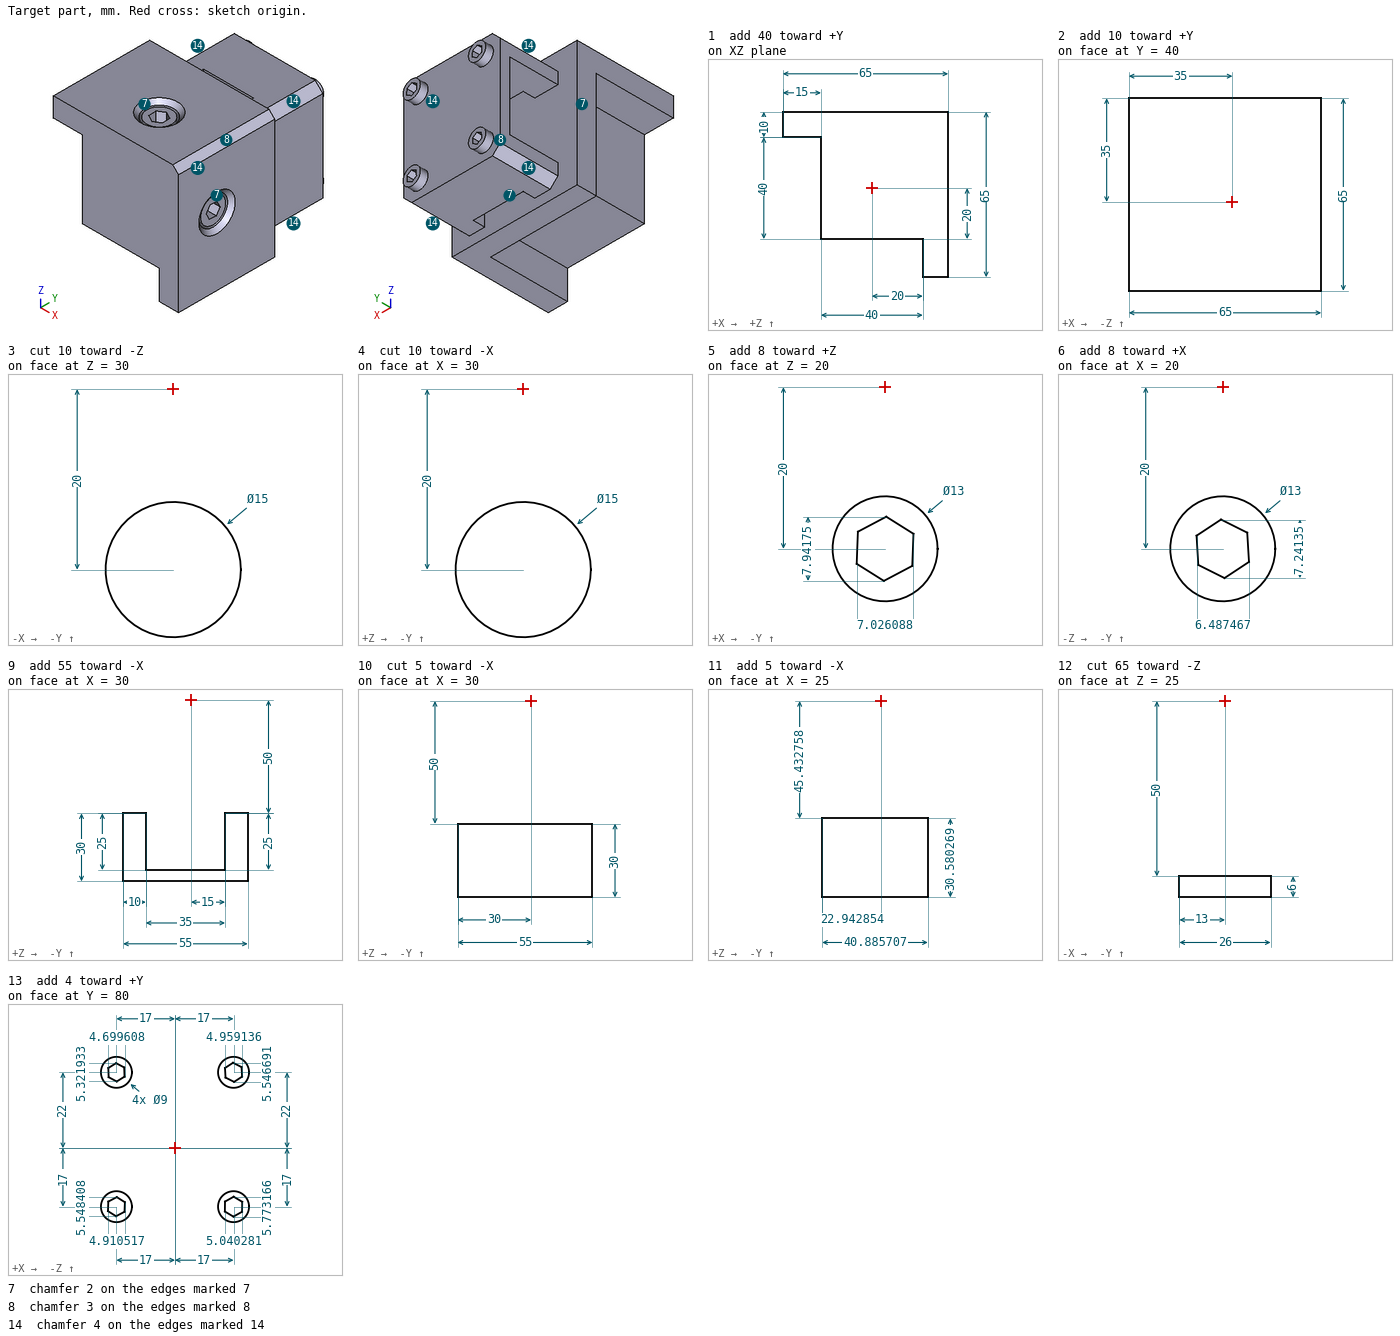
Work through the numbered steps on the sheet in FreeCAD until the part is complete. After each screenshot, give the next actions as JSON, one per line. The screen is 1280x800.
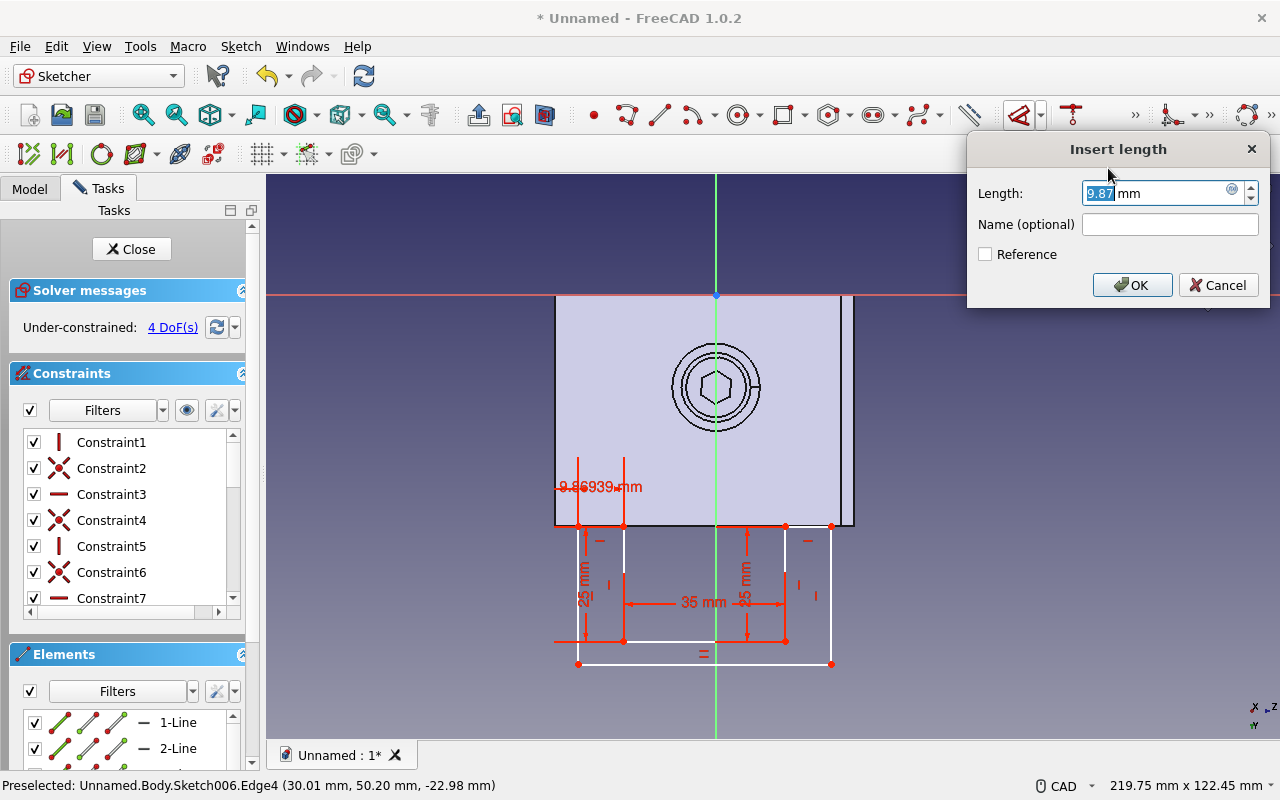
{"action": "type", "text": "10"}
{"action": "key", "text": "Return"}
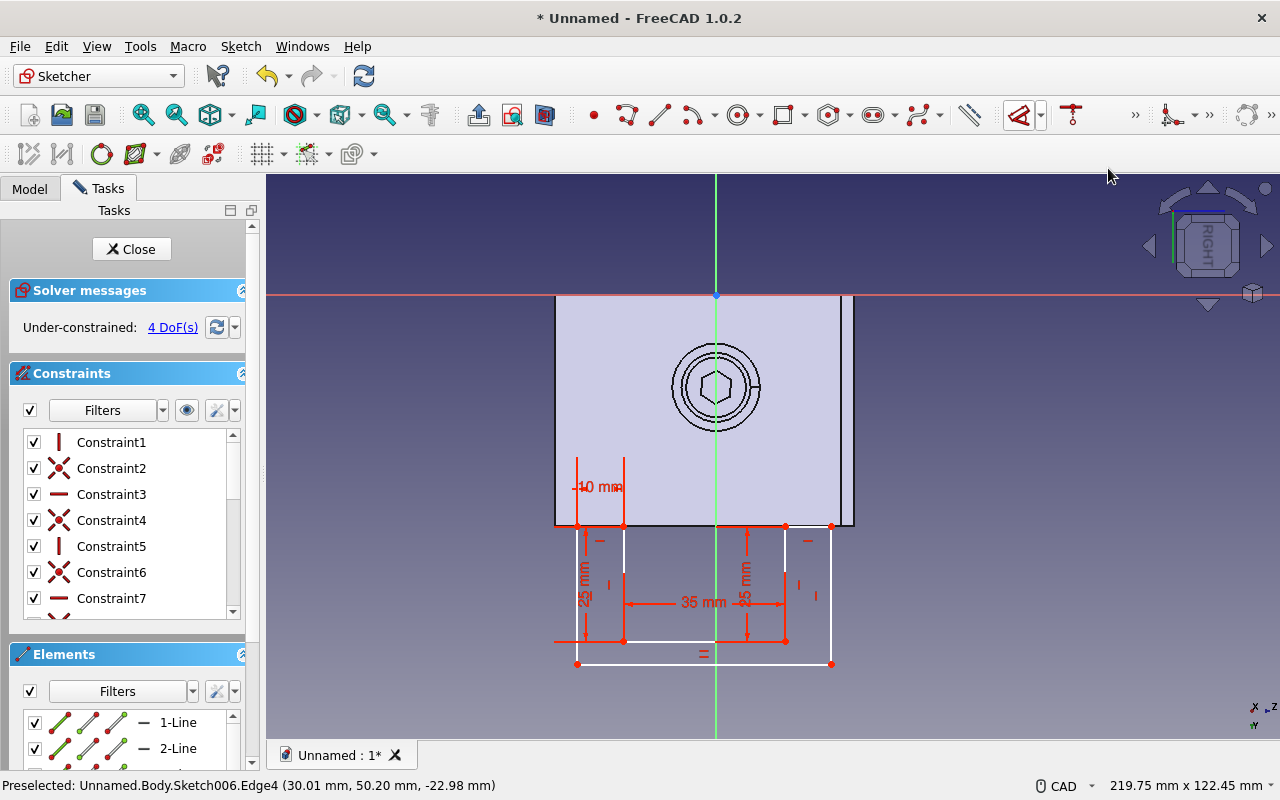
{"action": "left_click", "coordinate": [577, 568]}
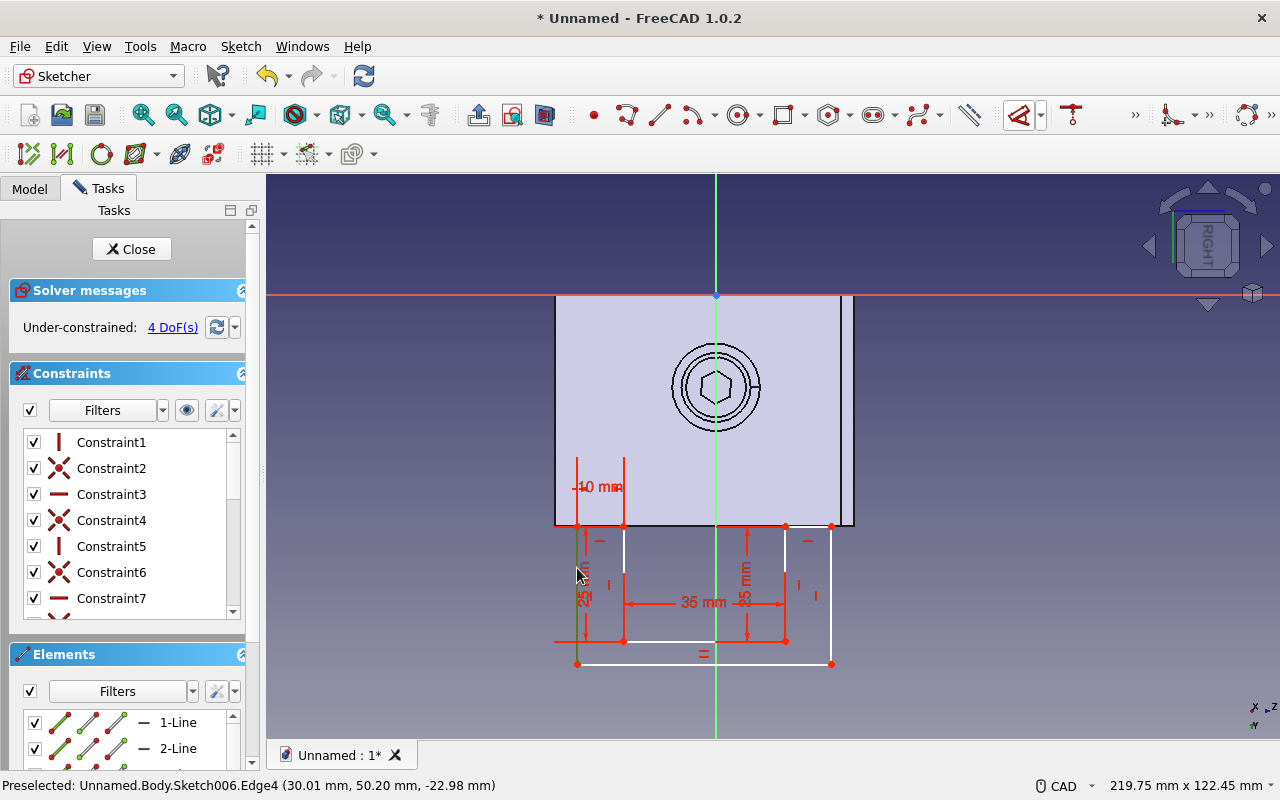
{"action": "key", "text": "i"}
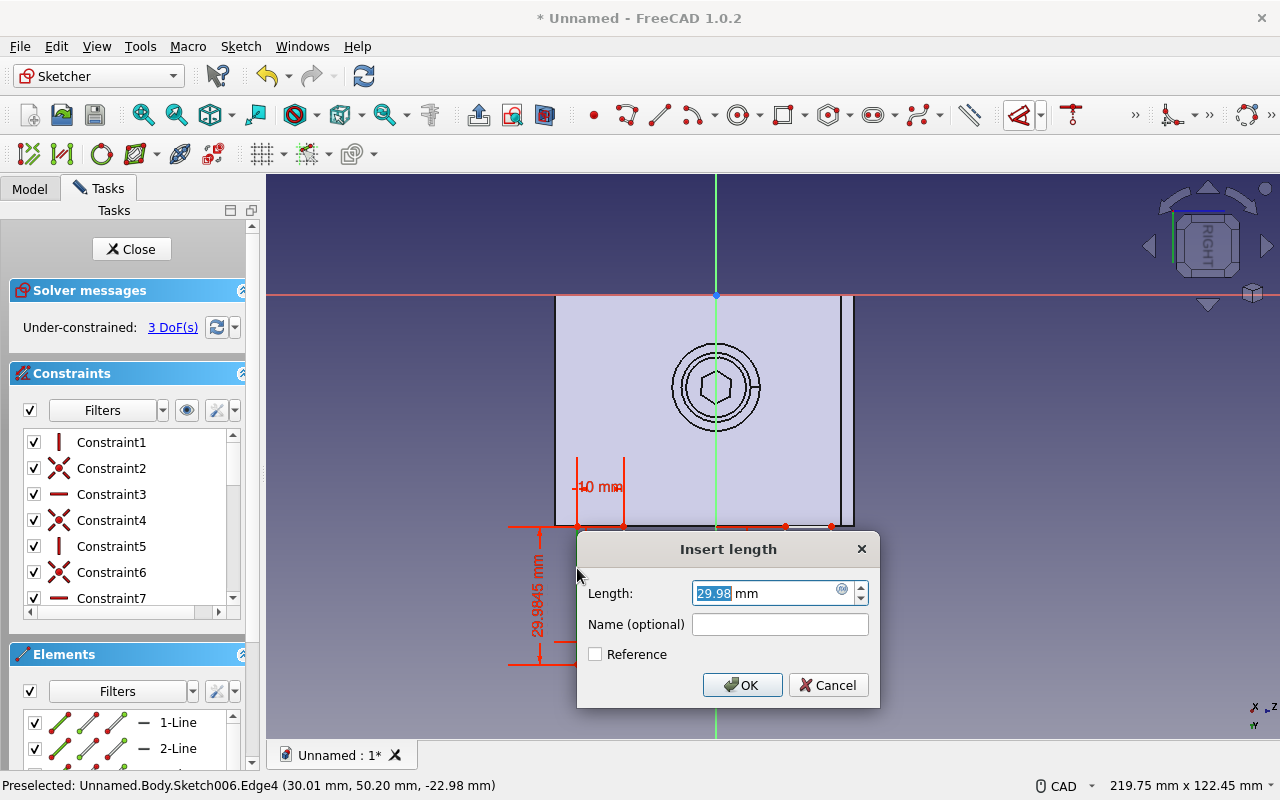
{"action": "type", "text": "30"}
{"action": "key", "text": "Return"}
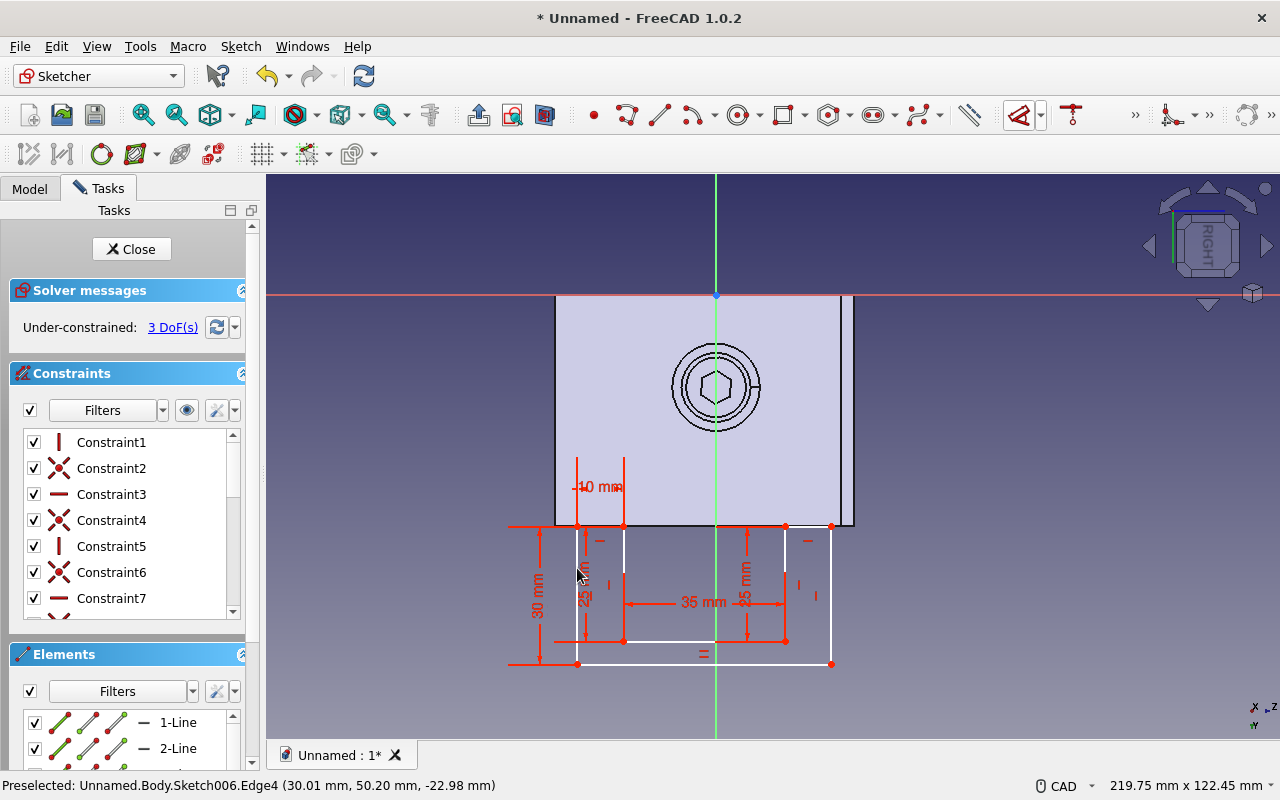
{"action": "left_click", "coordinate": [653, 665]}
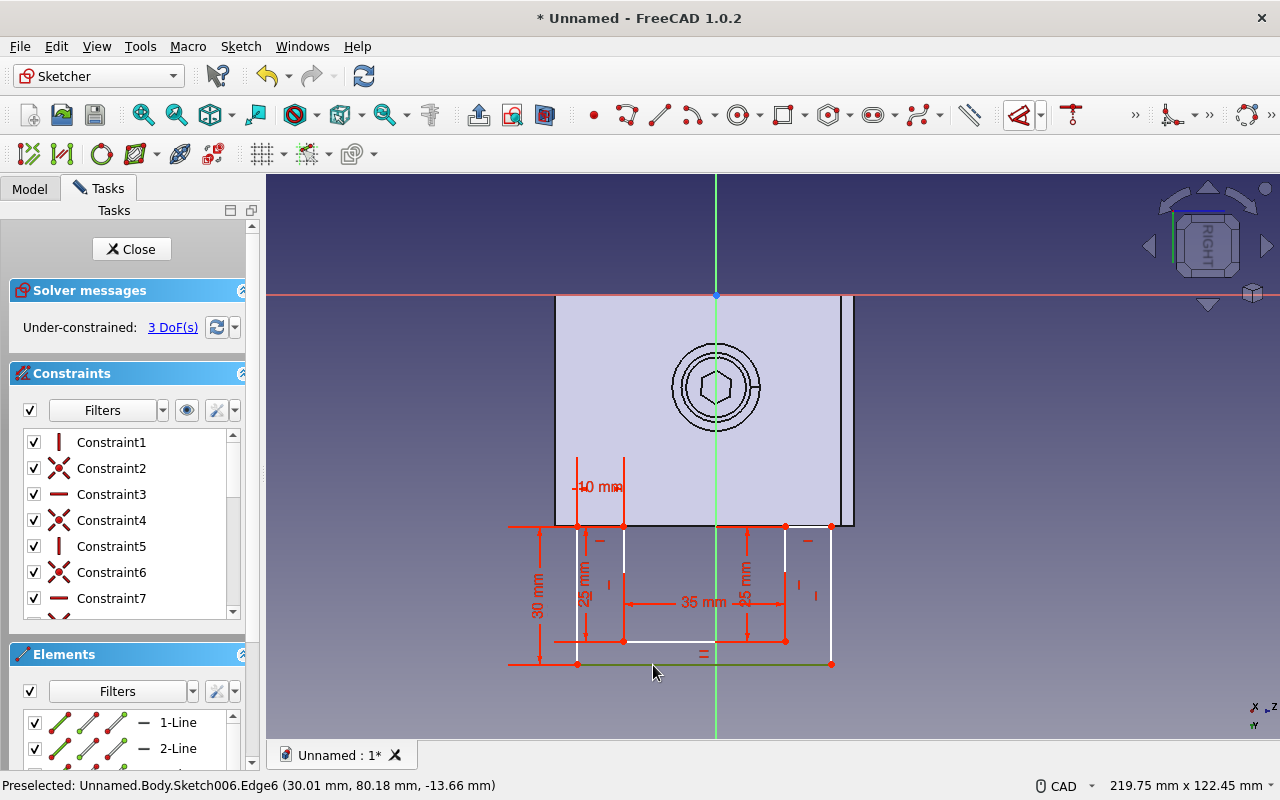
{"action": "left_click", "coordinate": [1040, 116]}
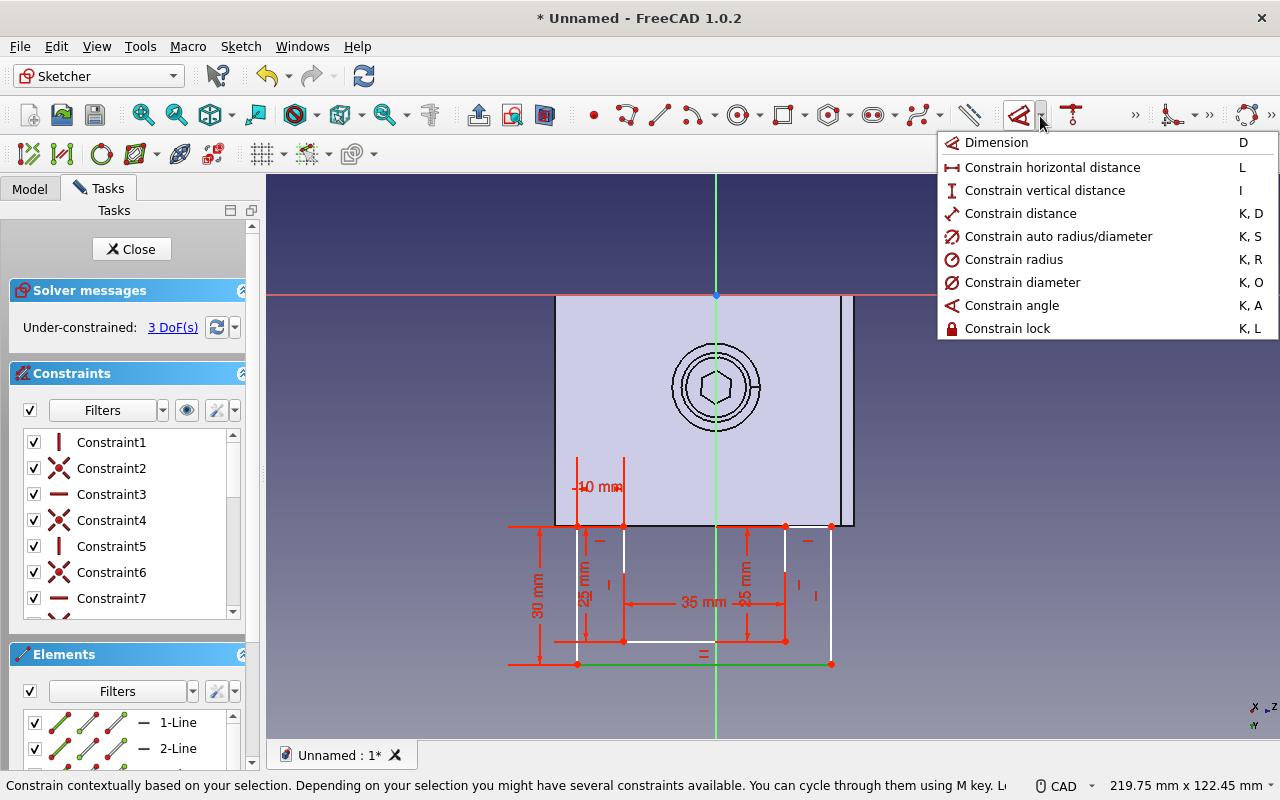
{"action": "left_click", "coordinate": [1108, 168]}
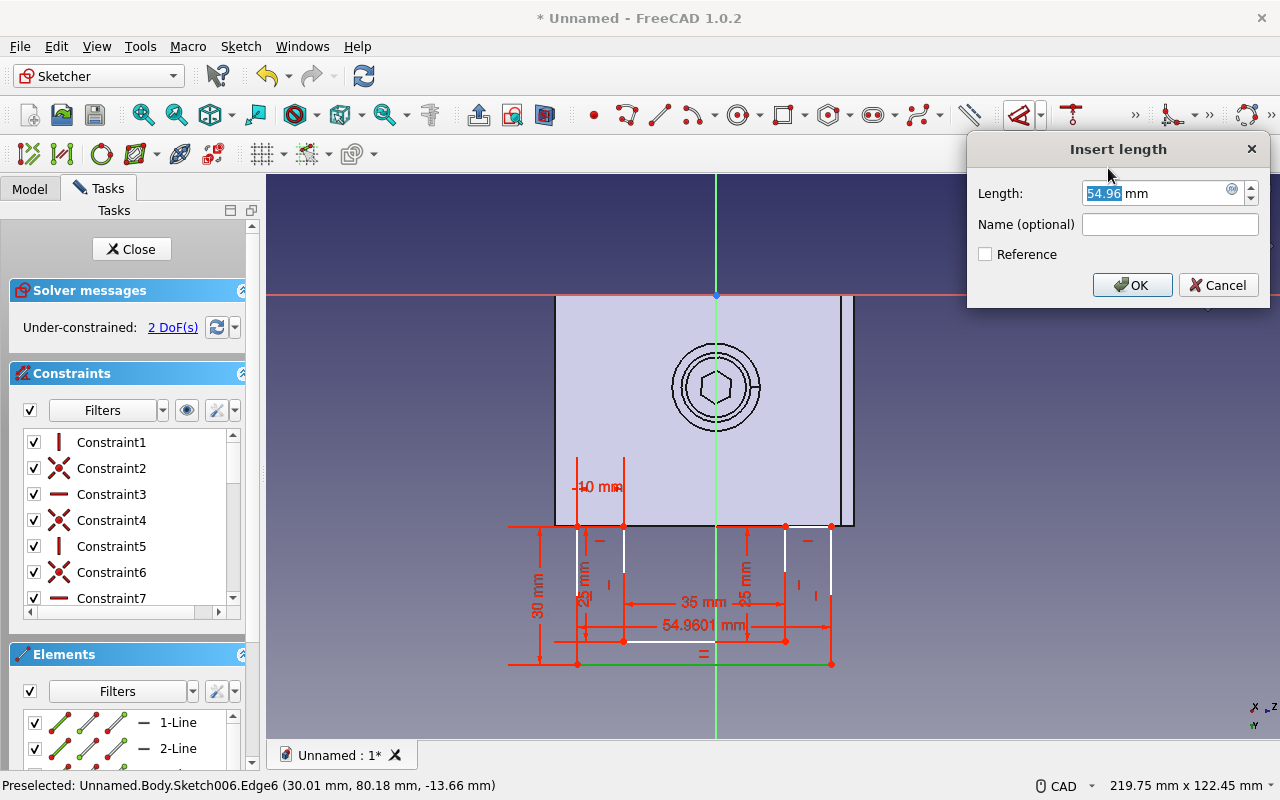
{"action": "type", "text": "55"}
{"action": "key", "text": "Return"}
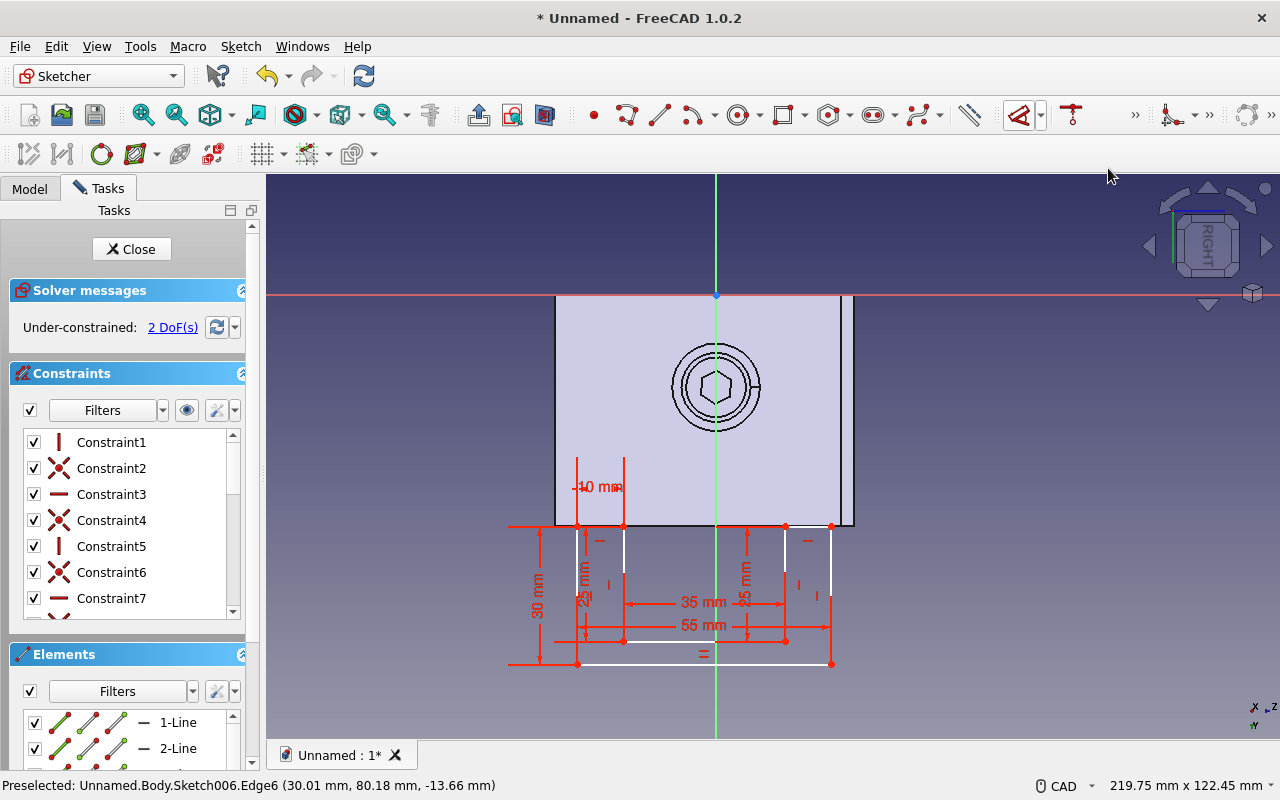
{"action": "left_click", "coordinate": [785, 527]}